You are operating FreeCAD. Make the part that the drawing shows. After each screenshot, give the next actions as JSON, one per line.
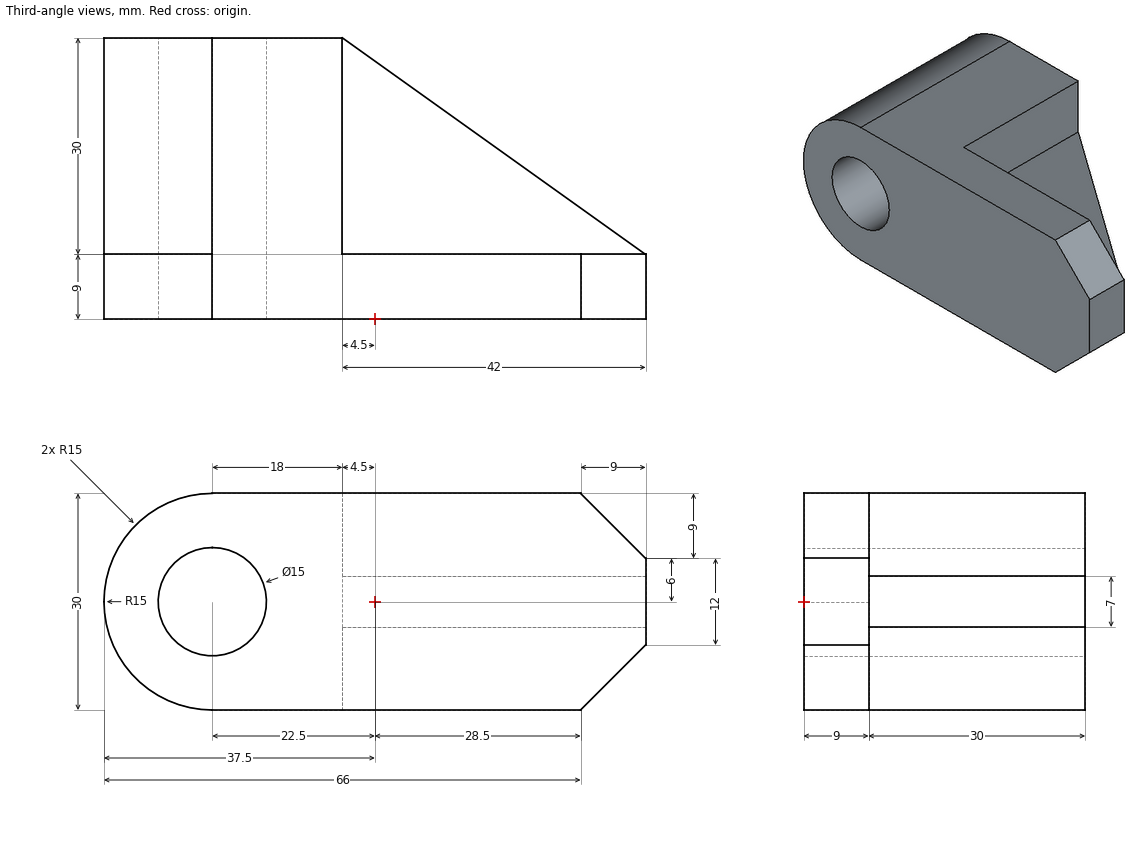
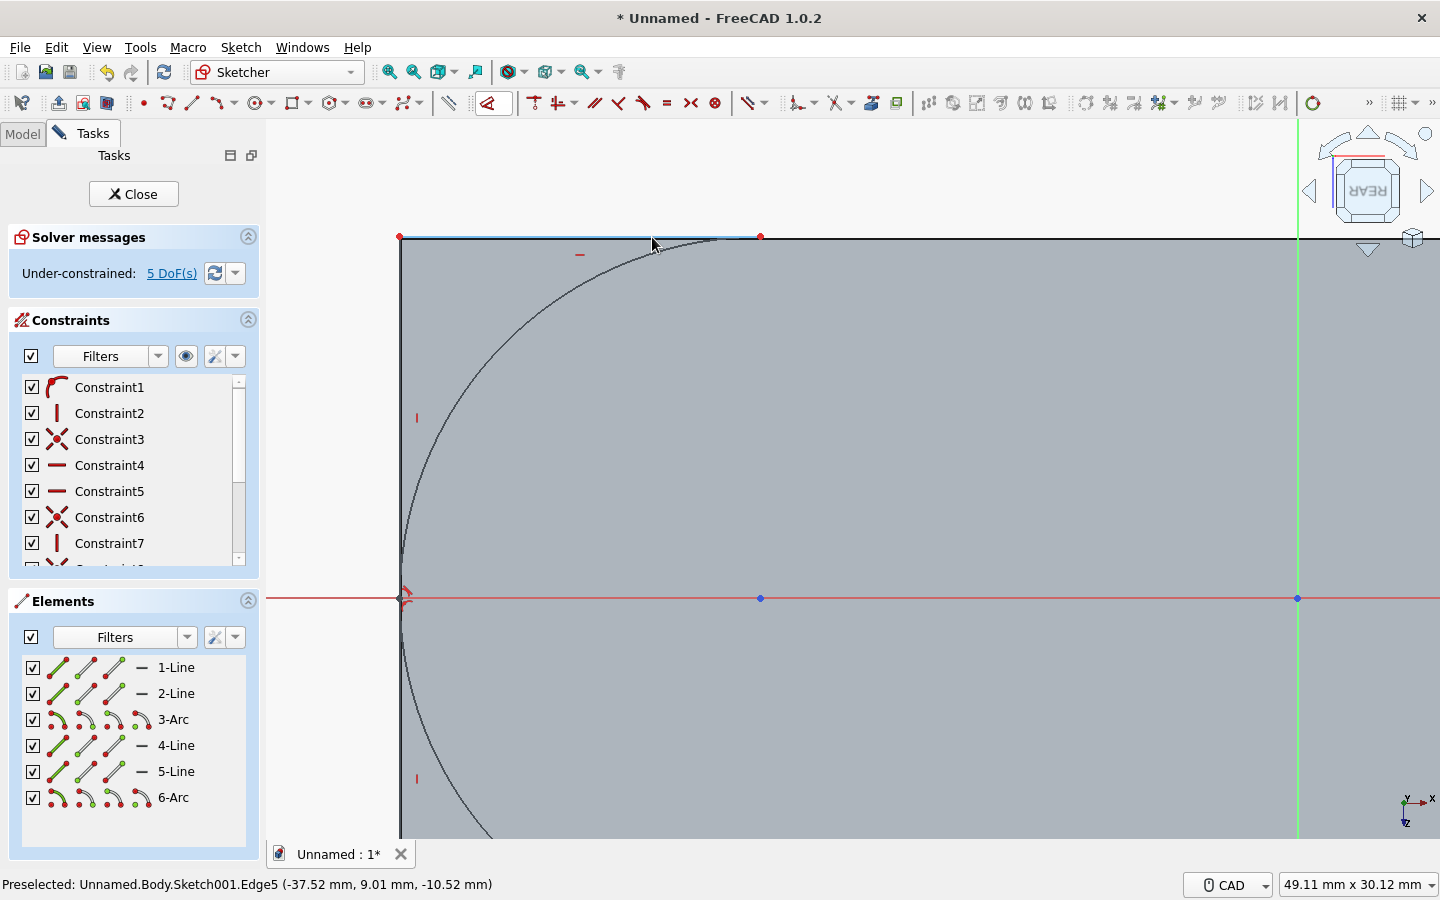
{"action": "left_click", "coordinate": [652, 237]}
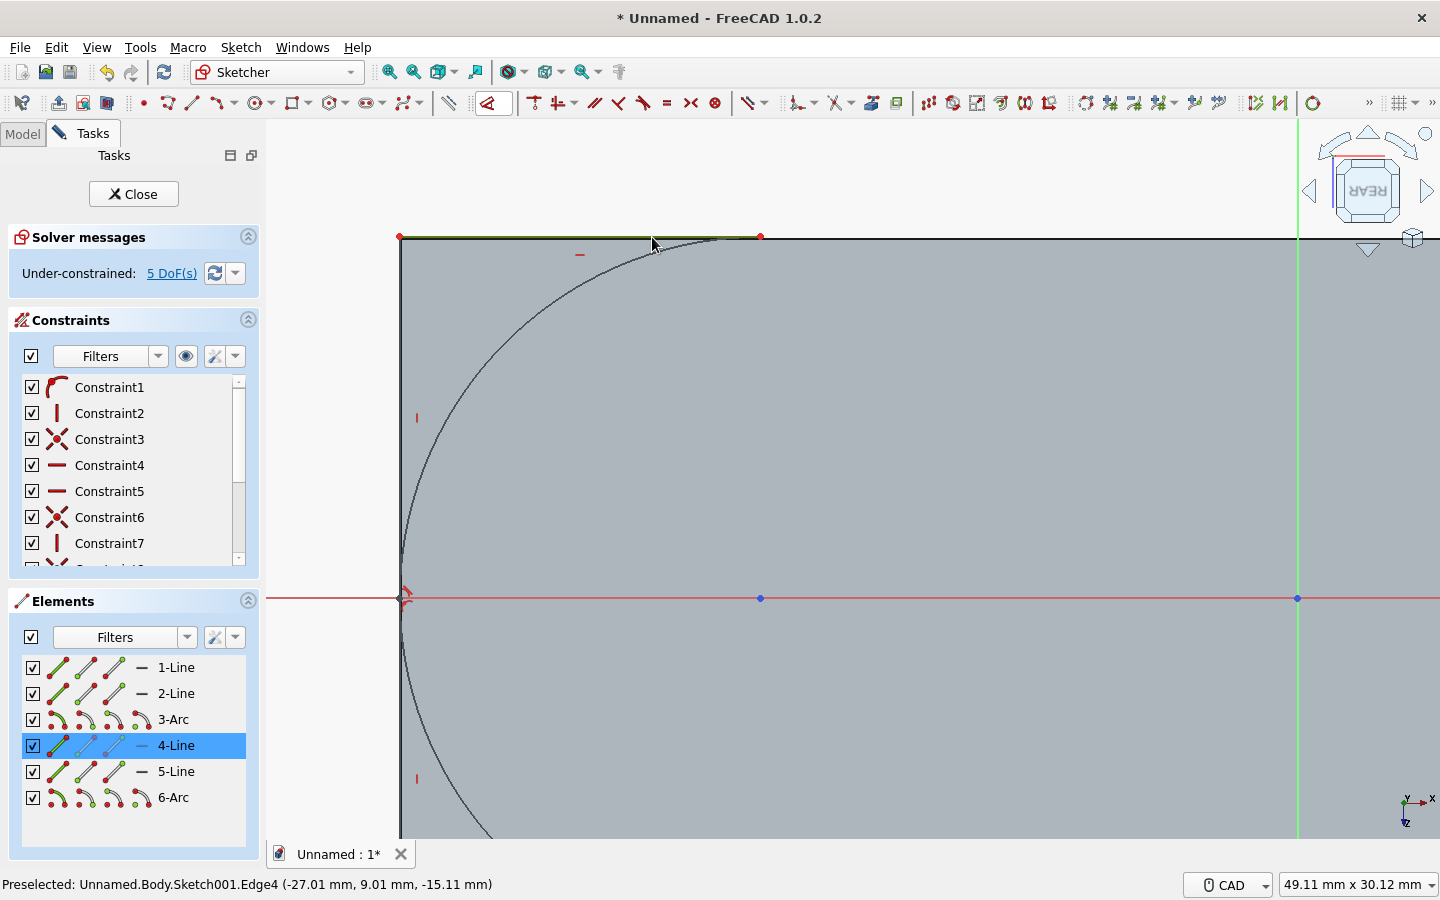
{"action": "left_click", "coordinate": [597, 276]}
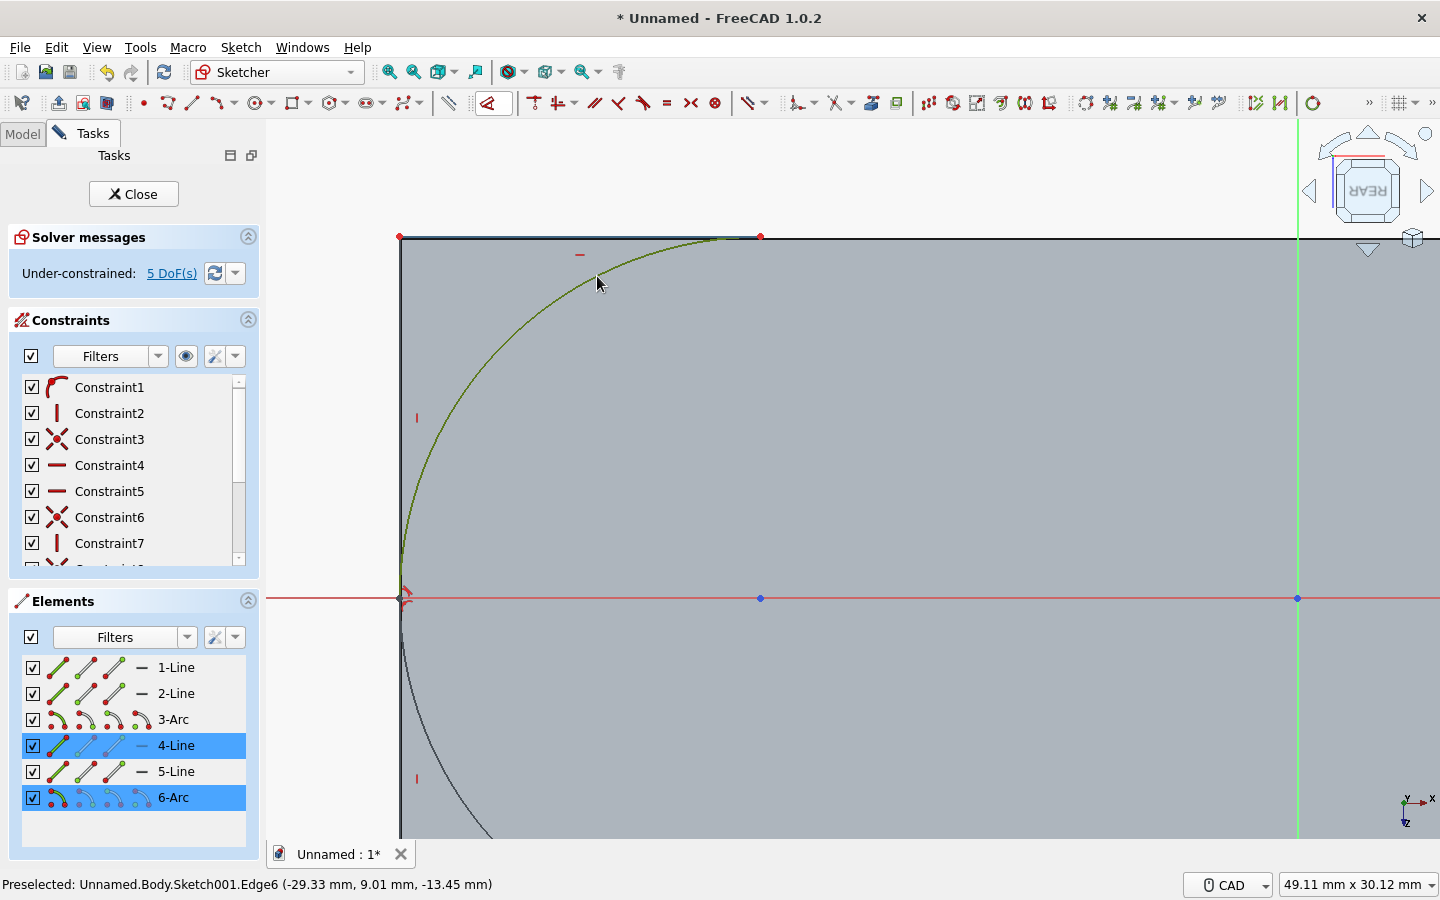
{"action": "key", "text": "t"}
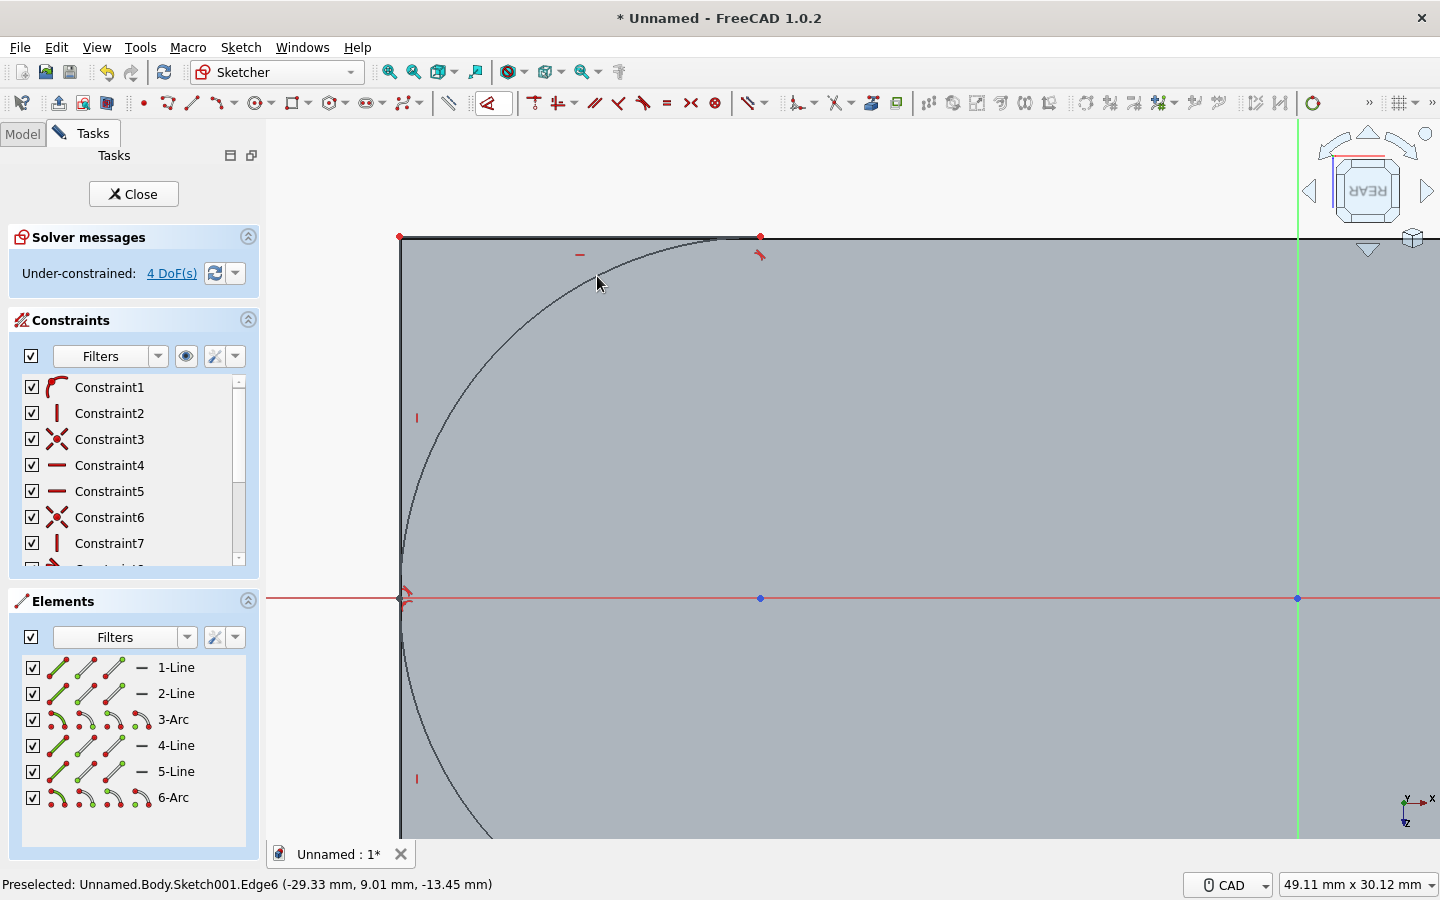
{"action": "left_click", "coordinate": [439, 762]}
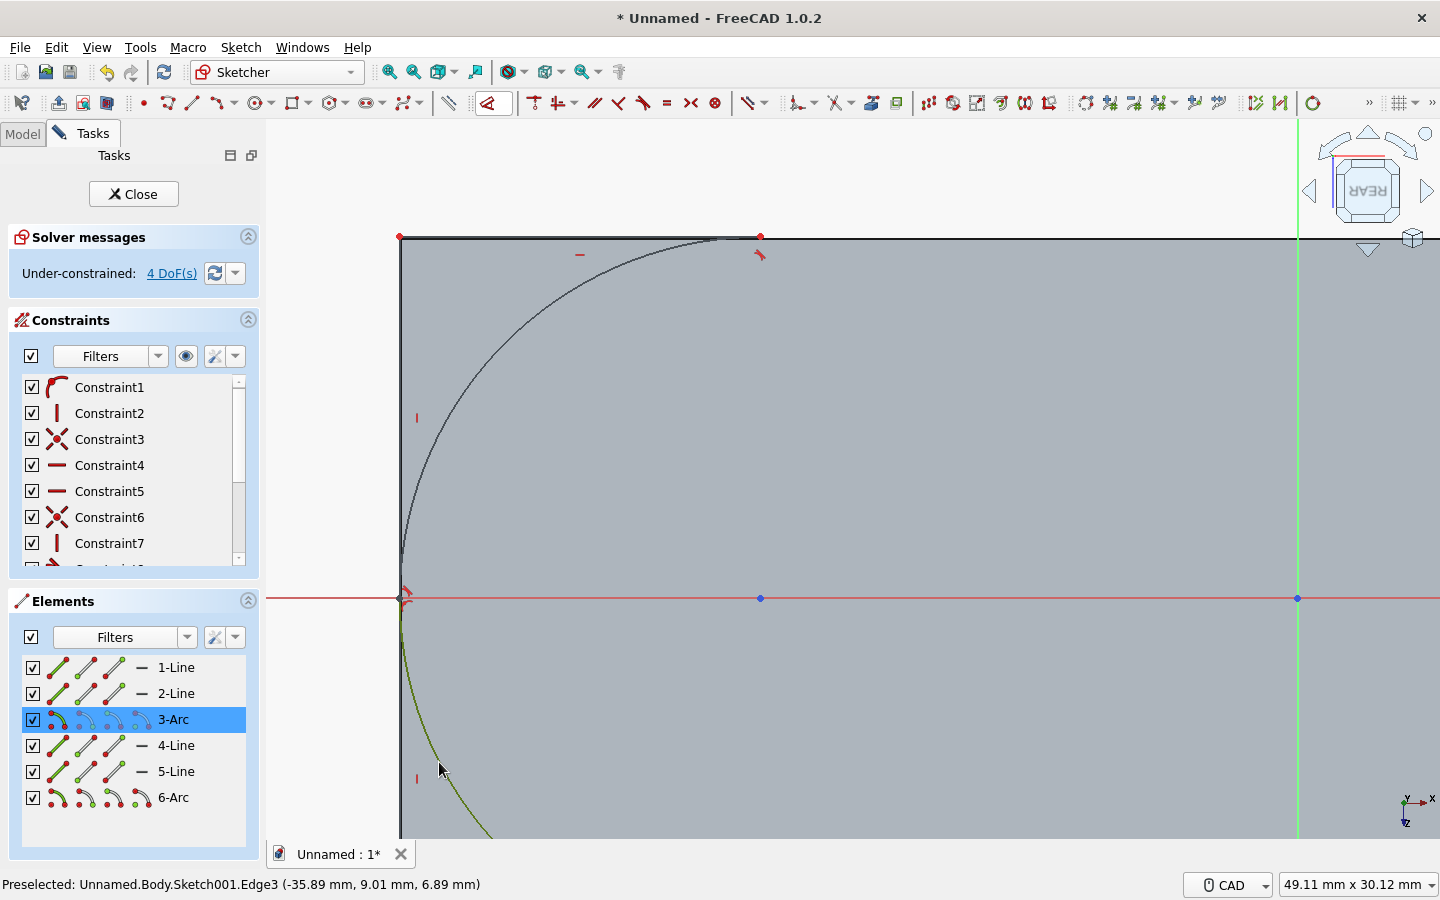
{"action": "left_click", "coordinate": [597, 276]}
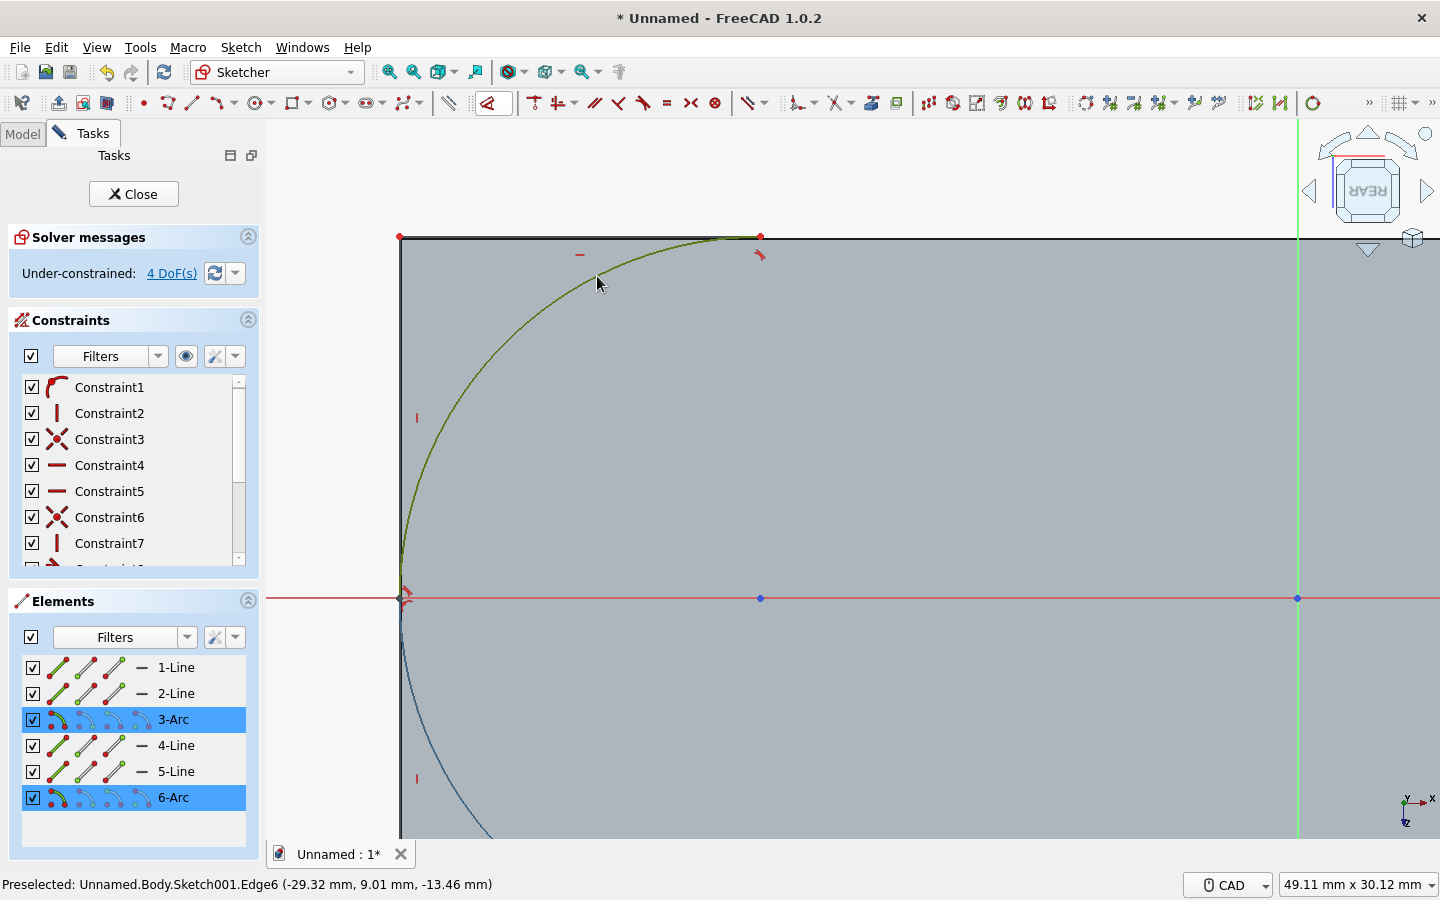
{"action": "key", "text": "e"}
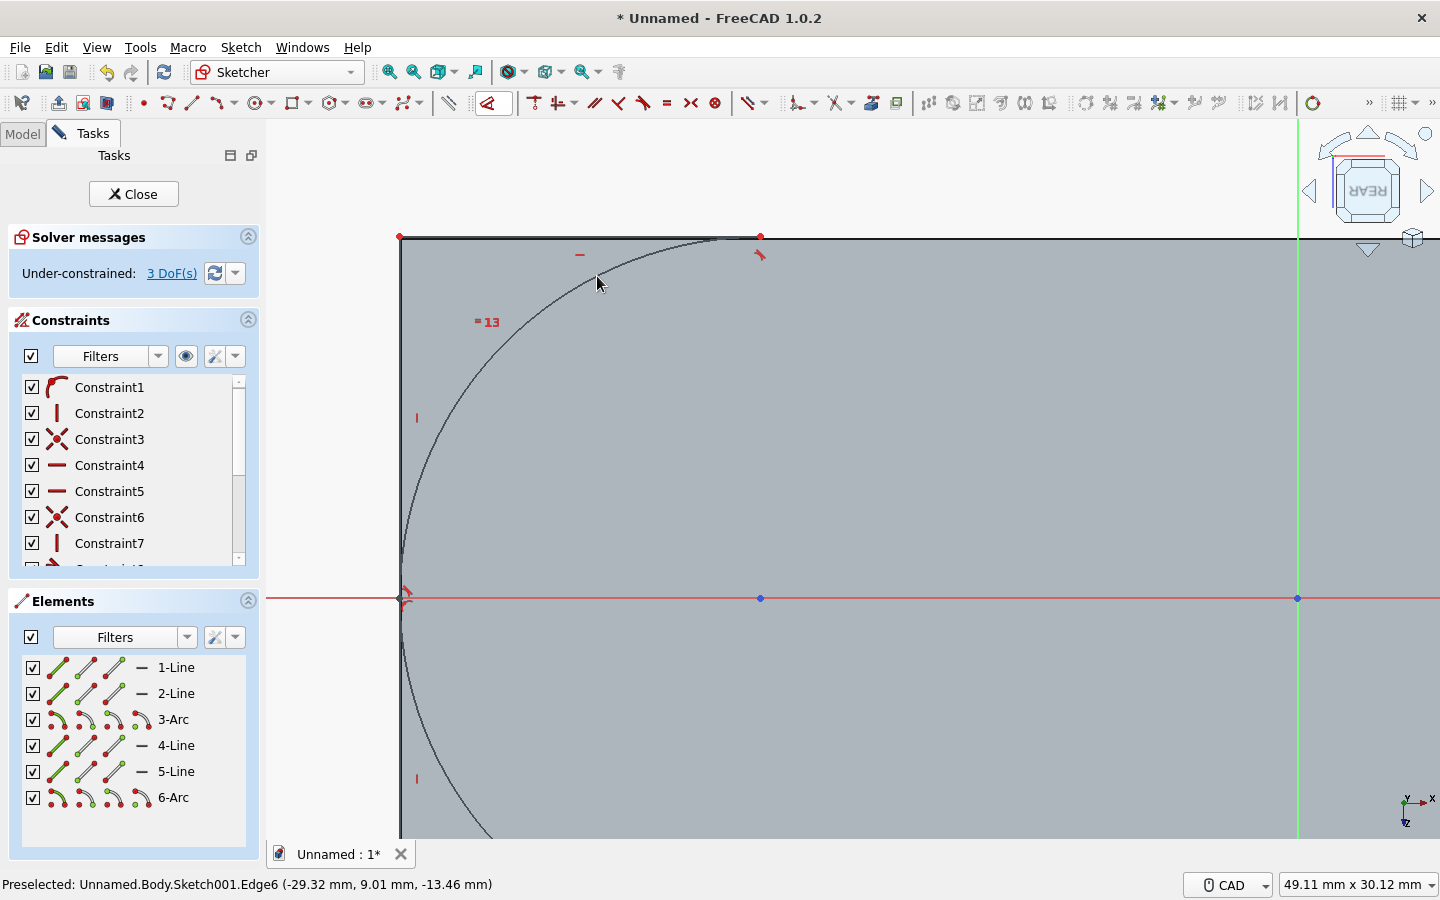
{"action": "left_click", "coordinate": [488, 104]}